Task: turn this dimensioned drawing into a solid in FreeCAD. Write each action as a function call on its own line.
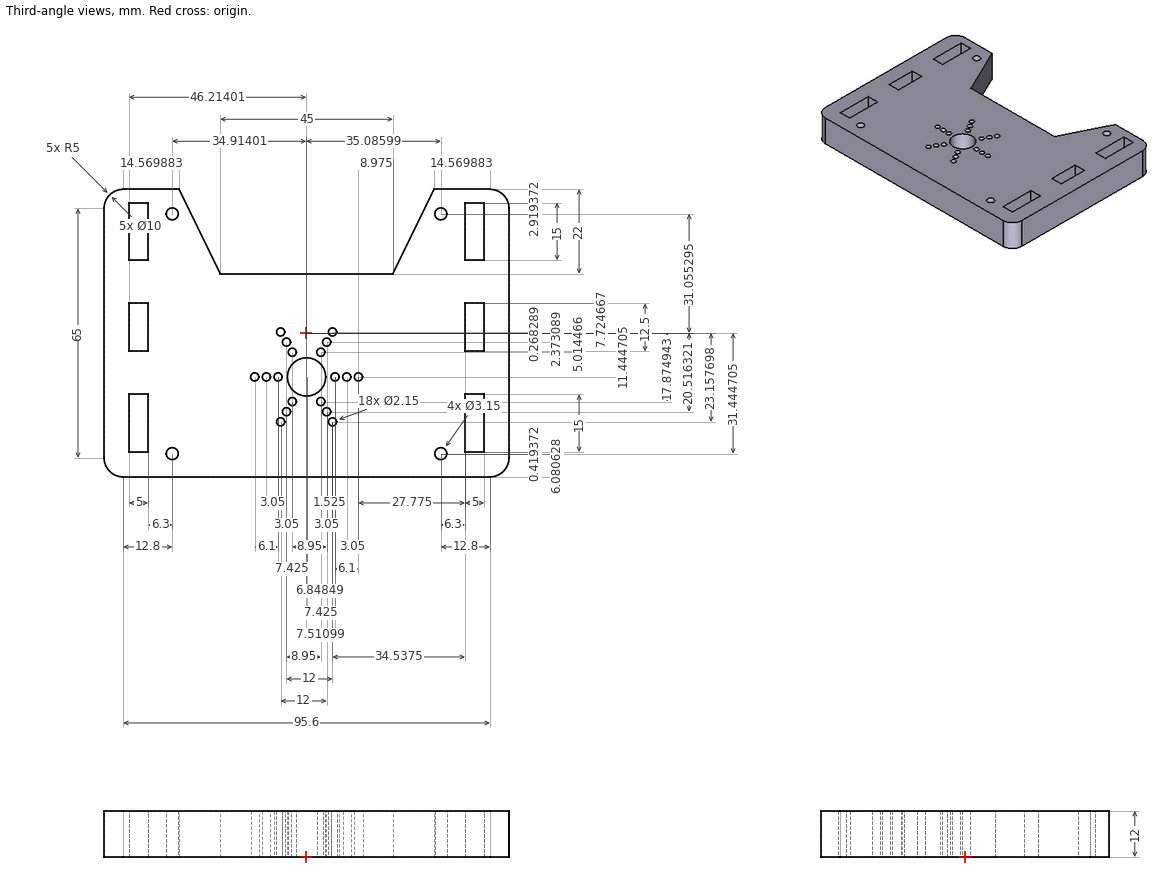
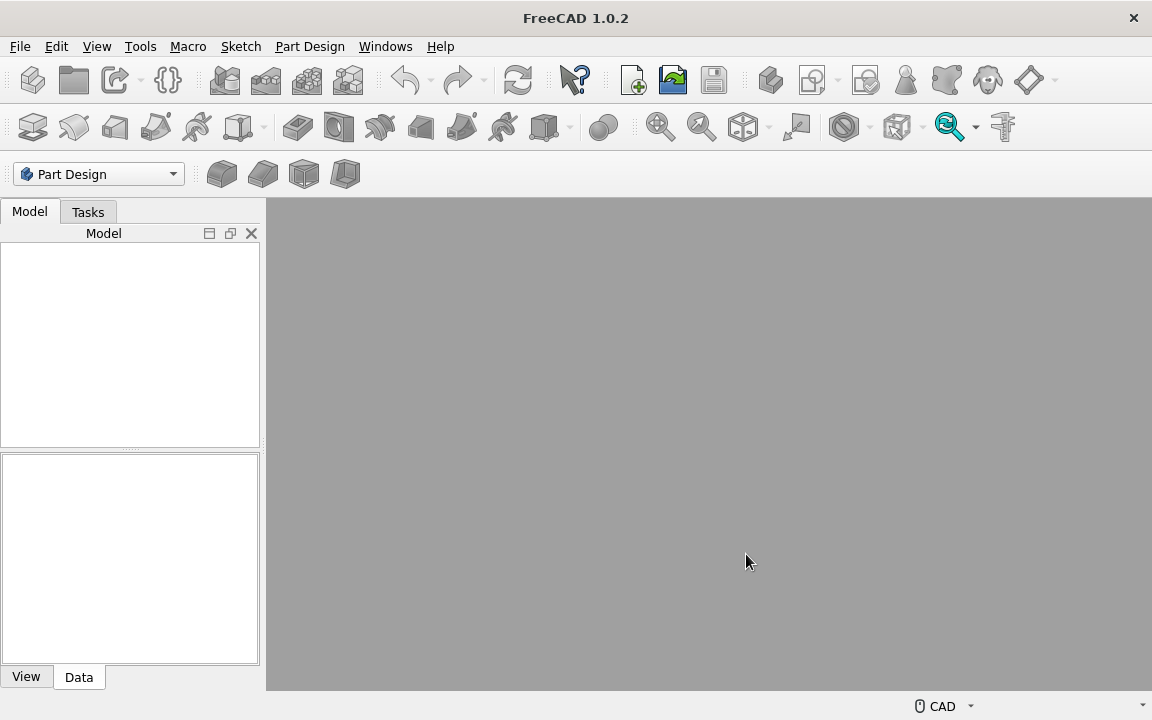
key(ctrl+n)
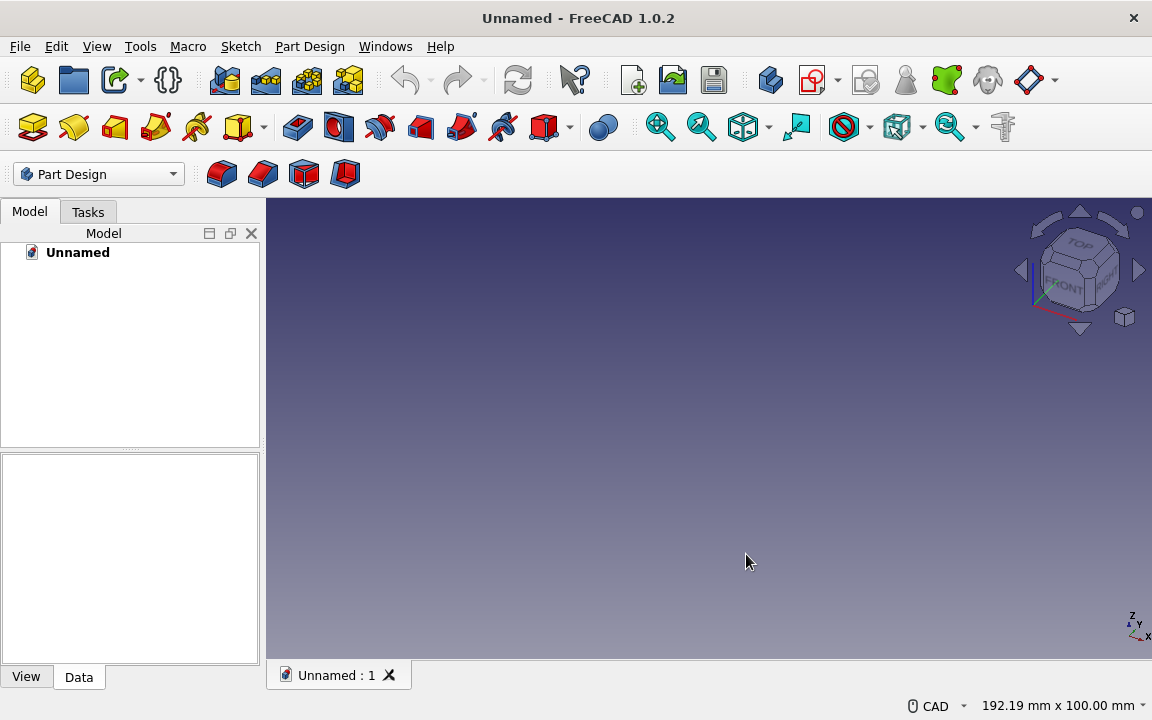
click(812, 80)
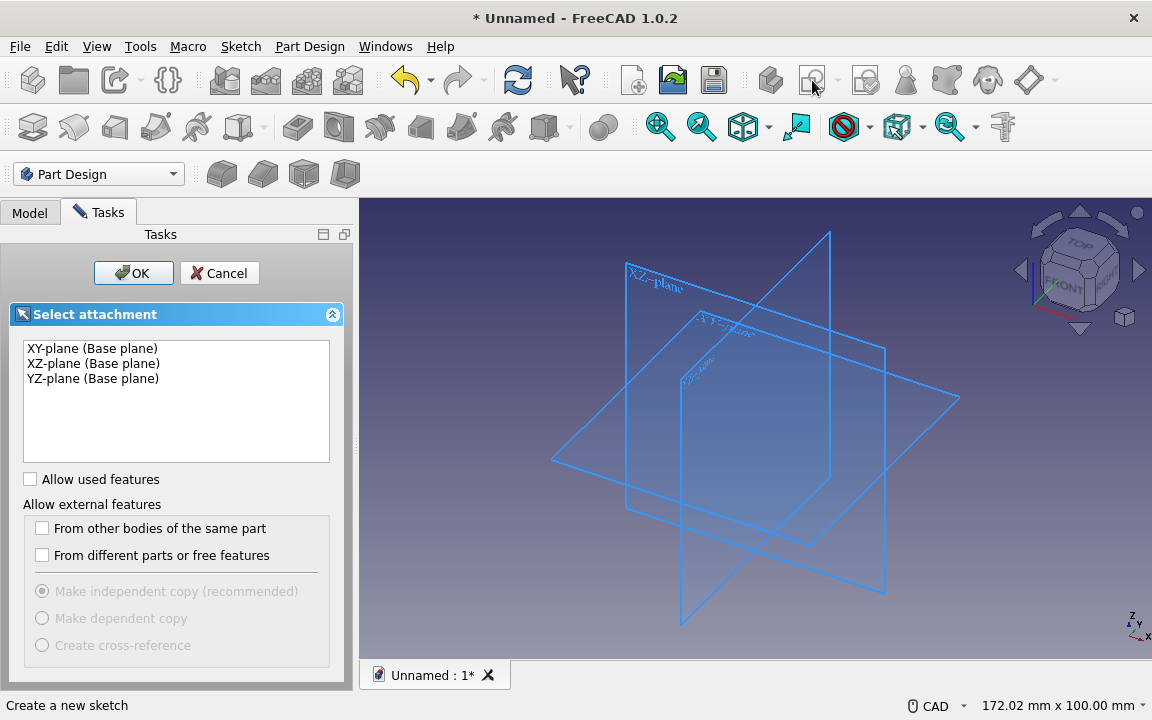
click(84, 348)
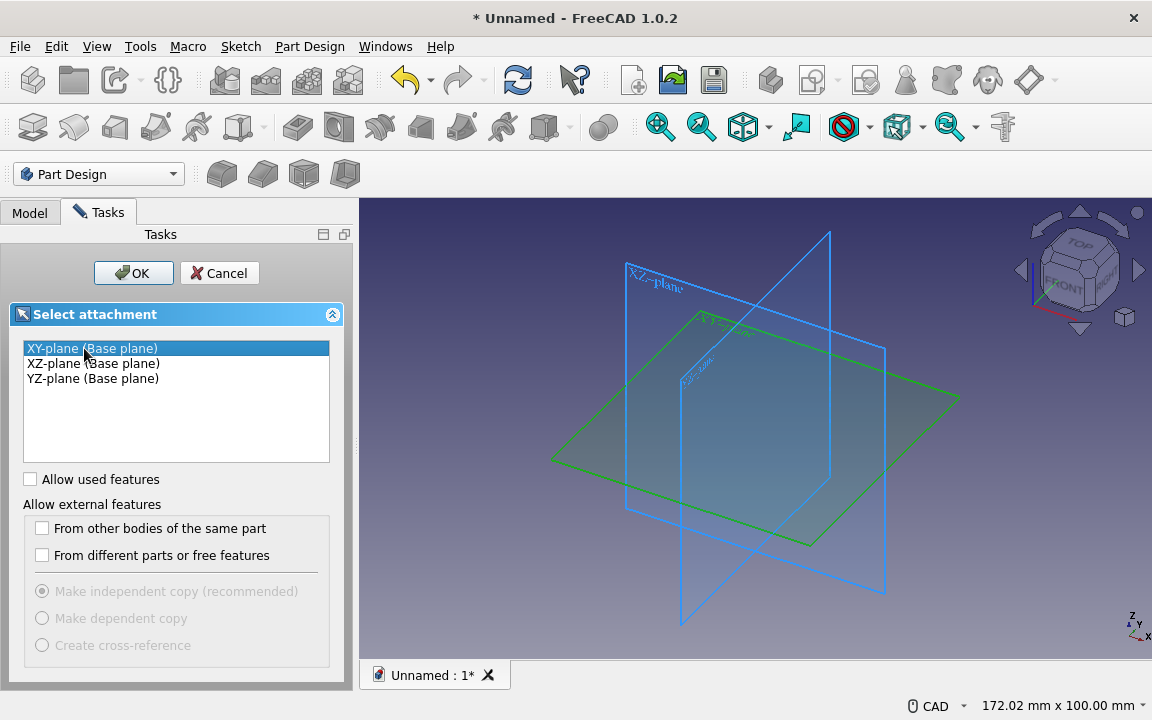
click(134, 273)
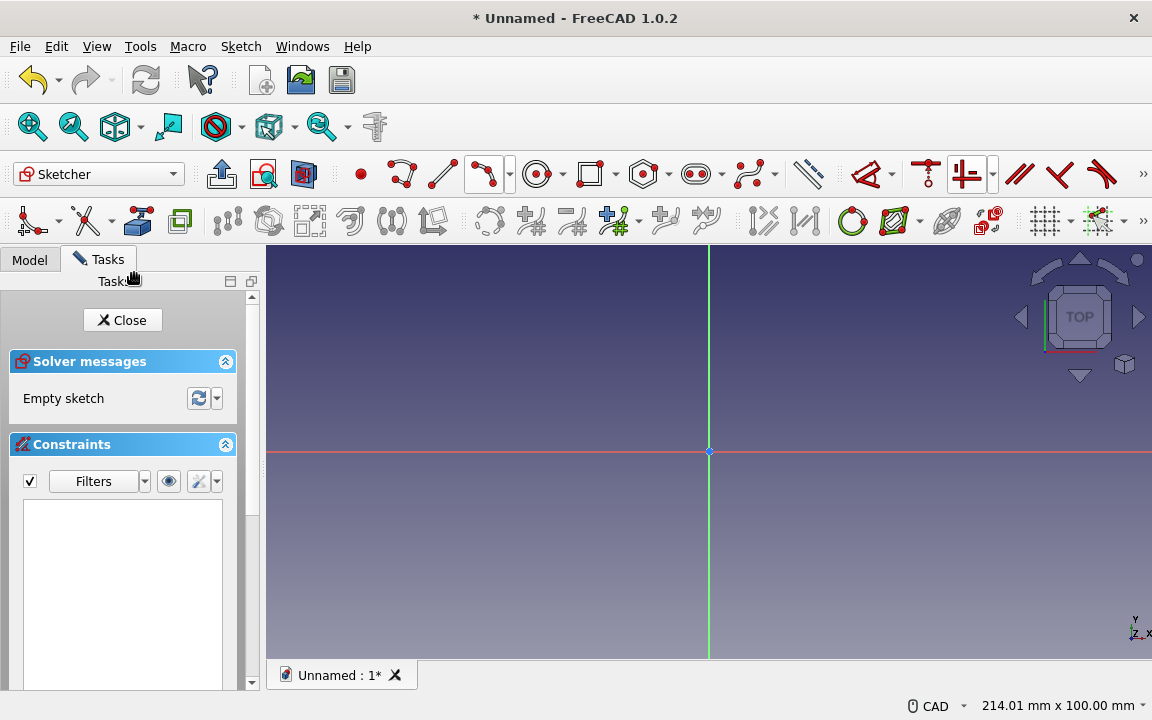
scroll(330, 452, down, 1)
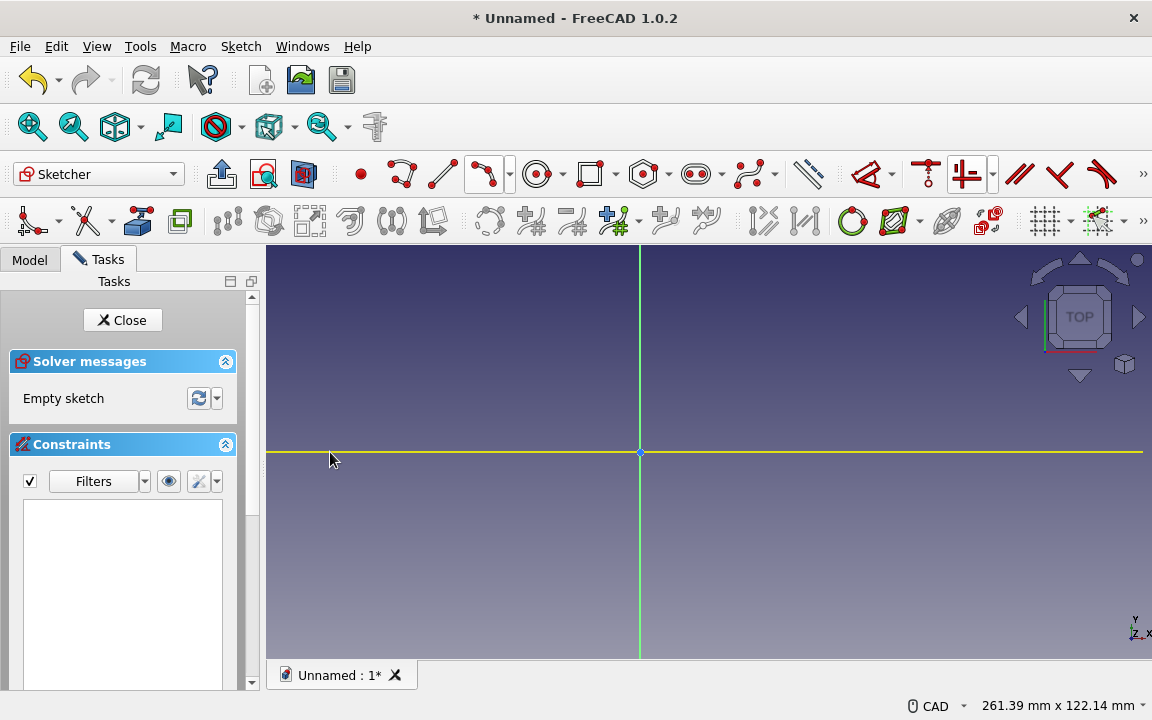
key(g)
key(l)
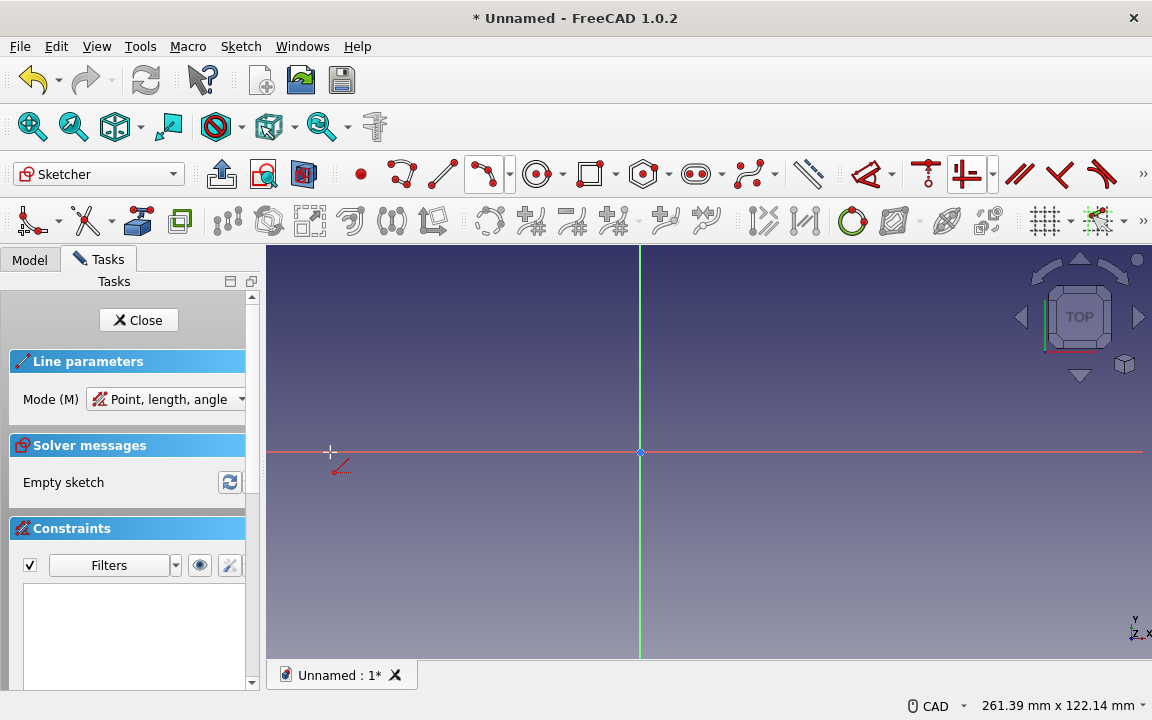
click(462, 342)
click(462, 562)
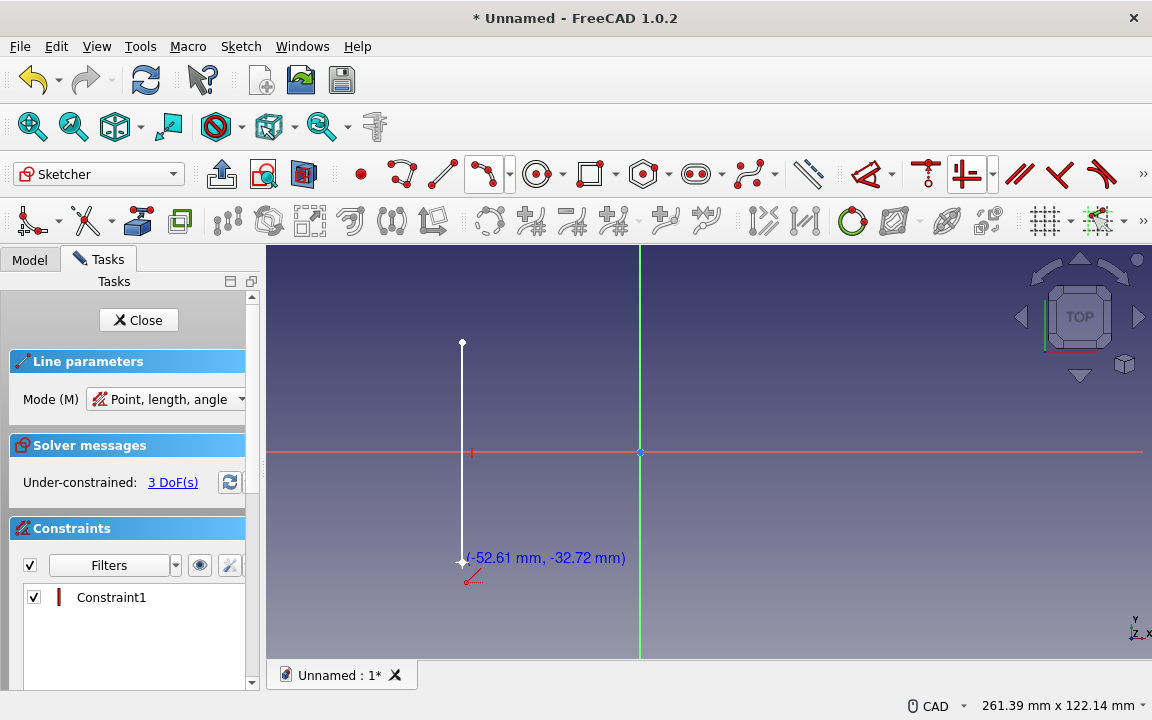
click(479, 579)
click(803, 579)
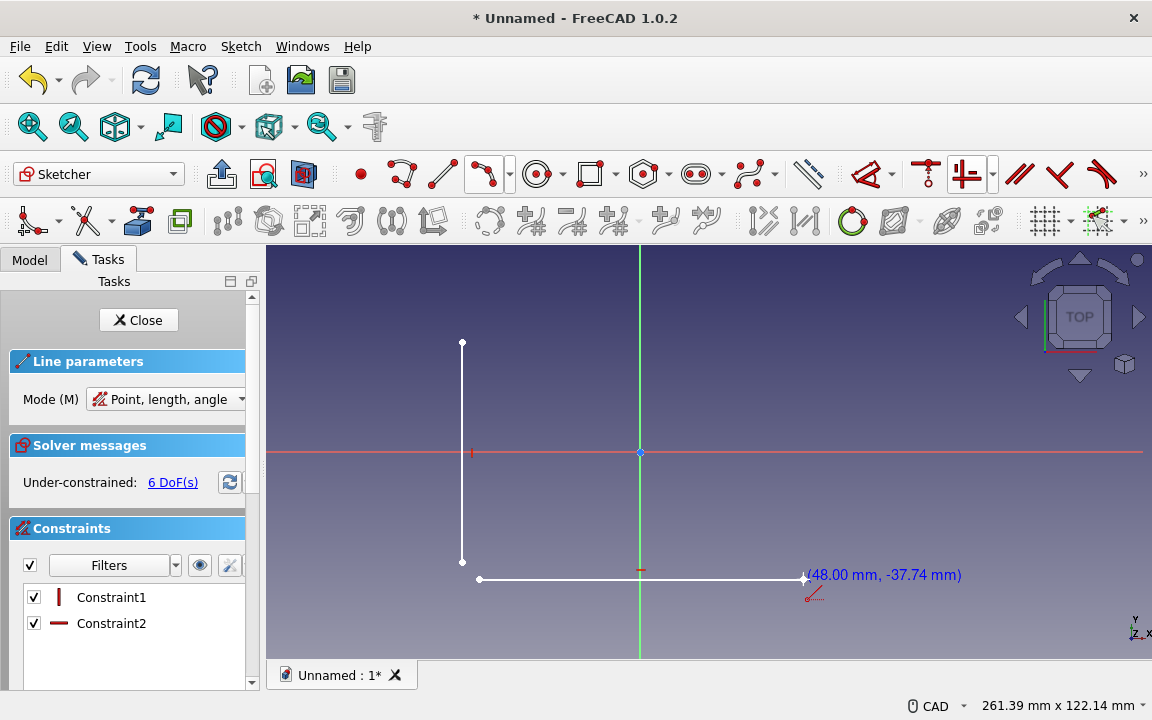
click(820, 562)
click(820, 342)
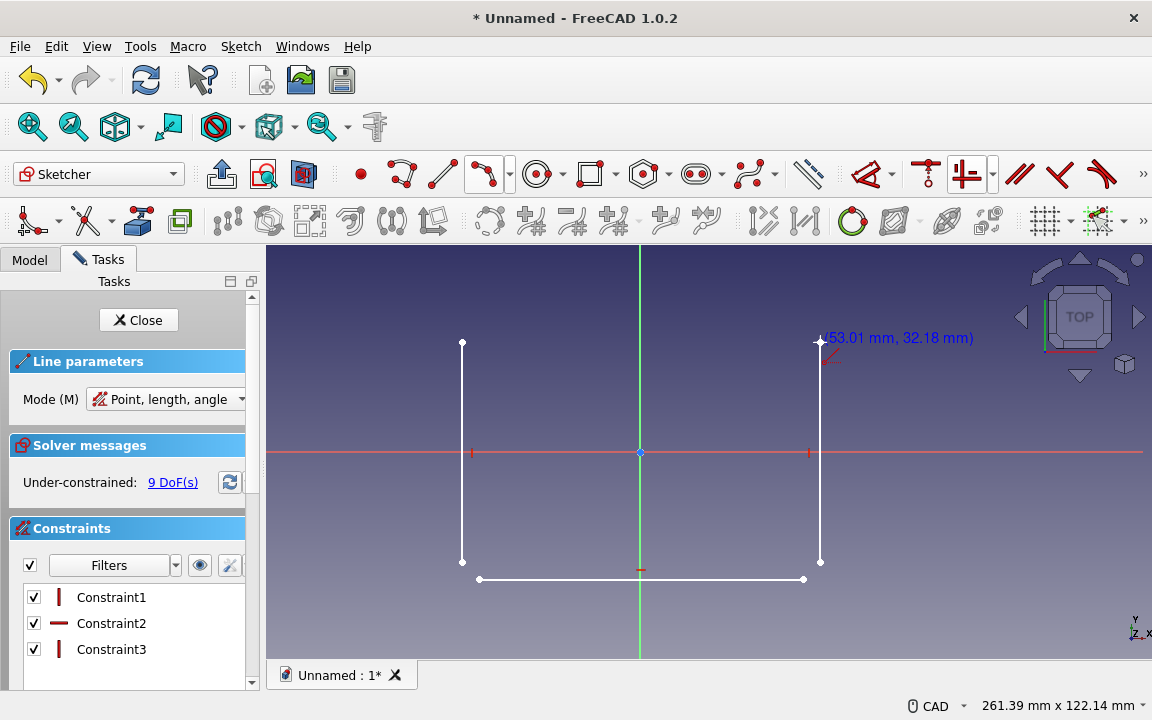
key(g)
key(m)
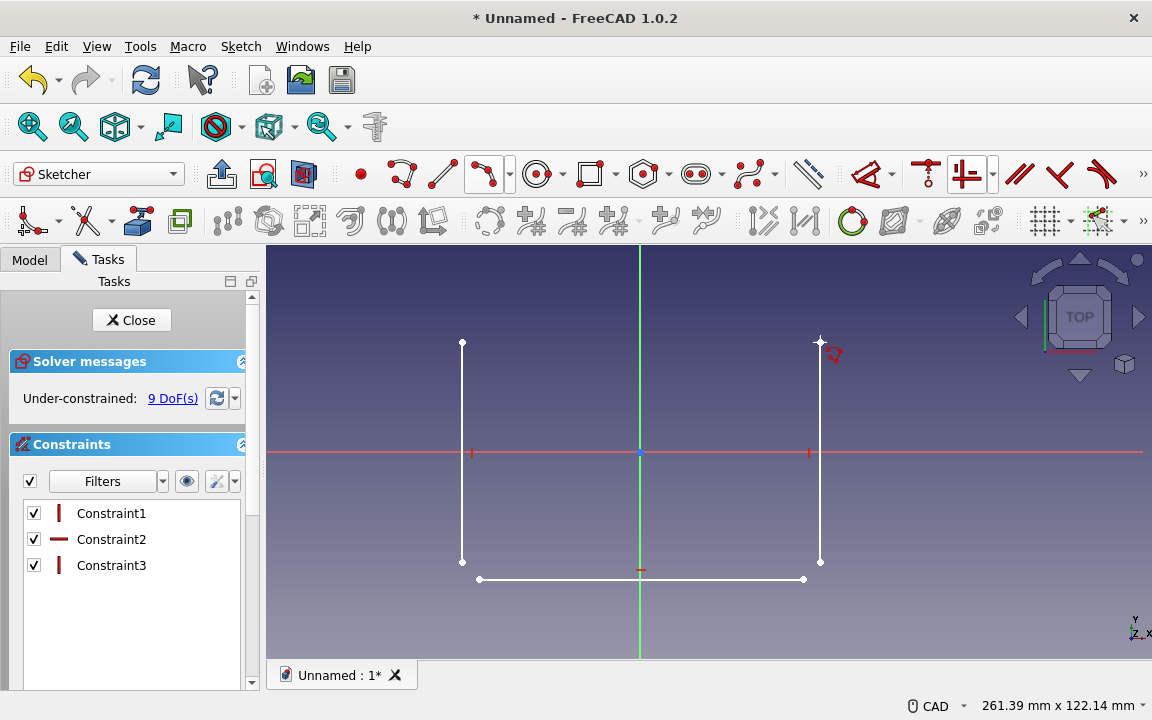
click(803, 325)
click(753, 325)
click(717, 400)
click(564, 400)
click(528, 325)
click(479, 325)
right_click(479, 325)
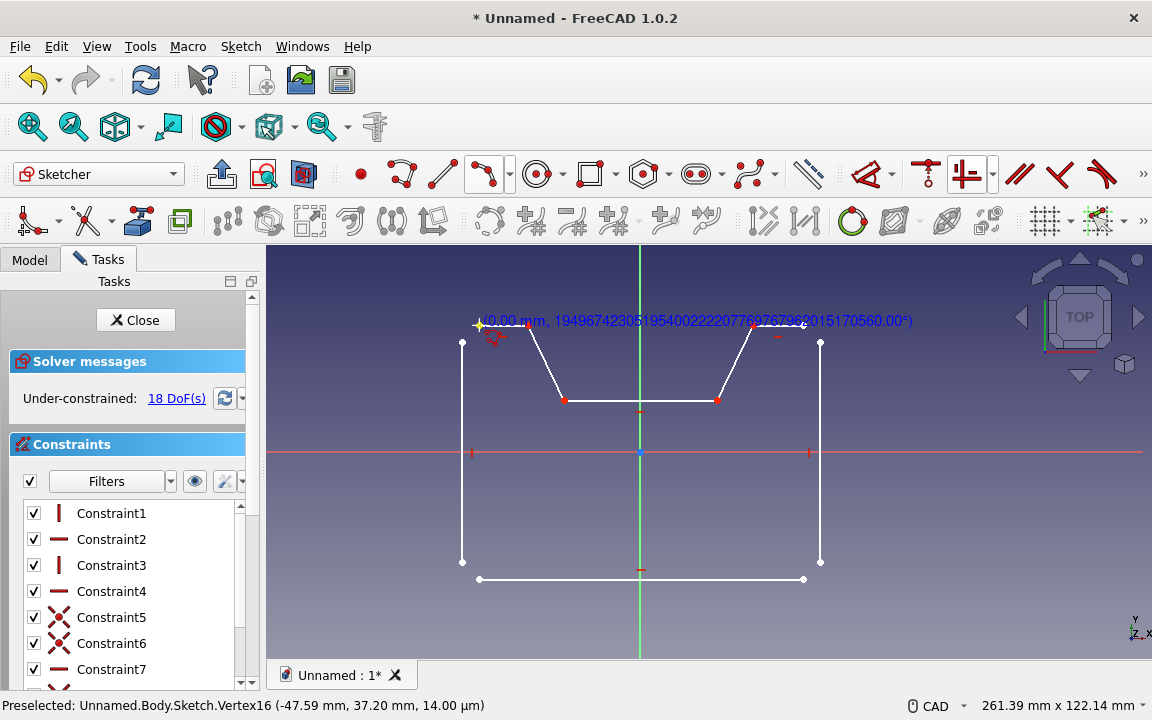
click(484, 174)